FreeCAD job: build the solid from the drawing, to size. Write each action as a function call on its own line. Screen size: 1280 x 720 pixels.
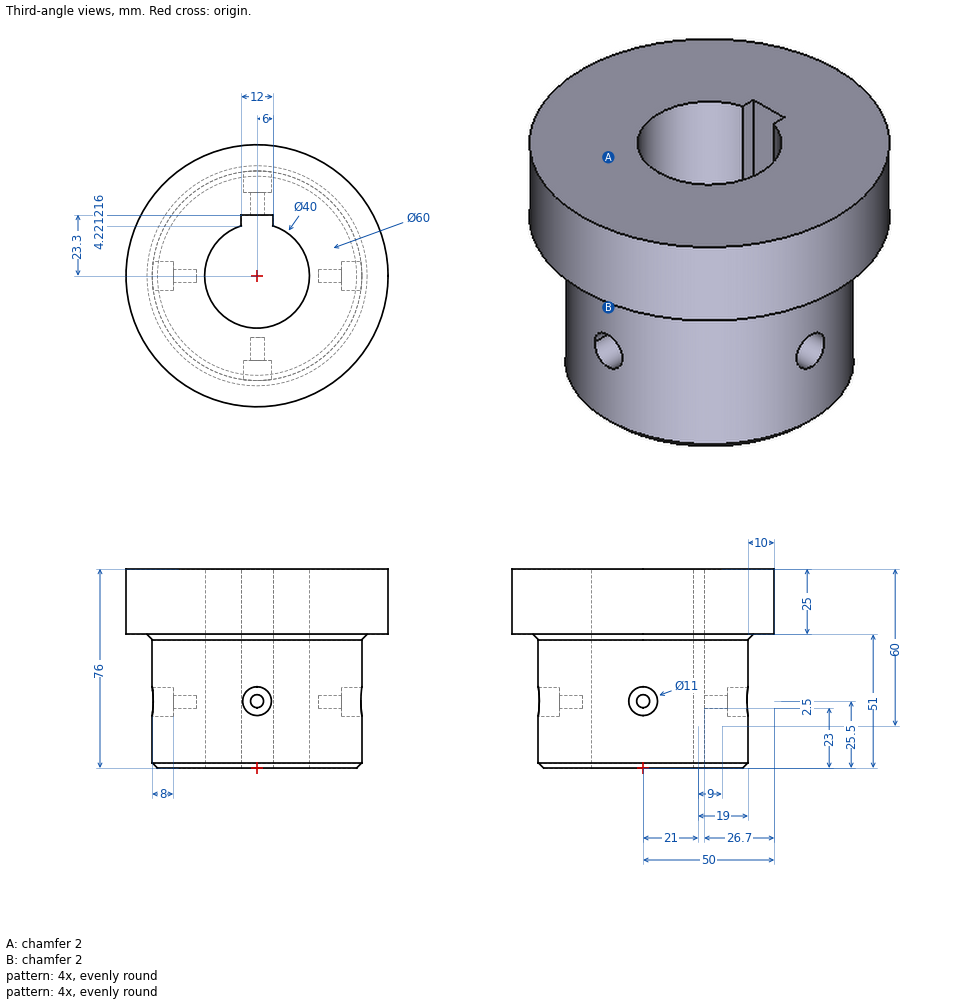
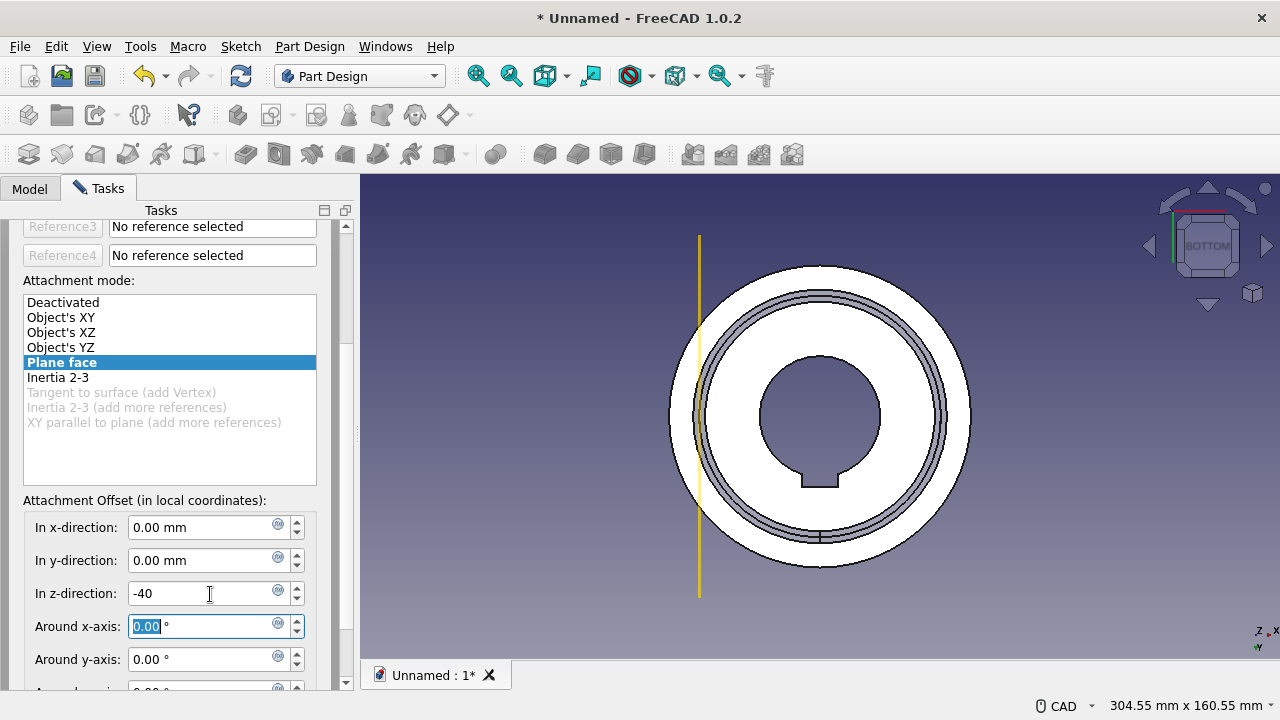
scroll(346, 455, up, 4)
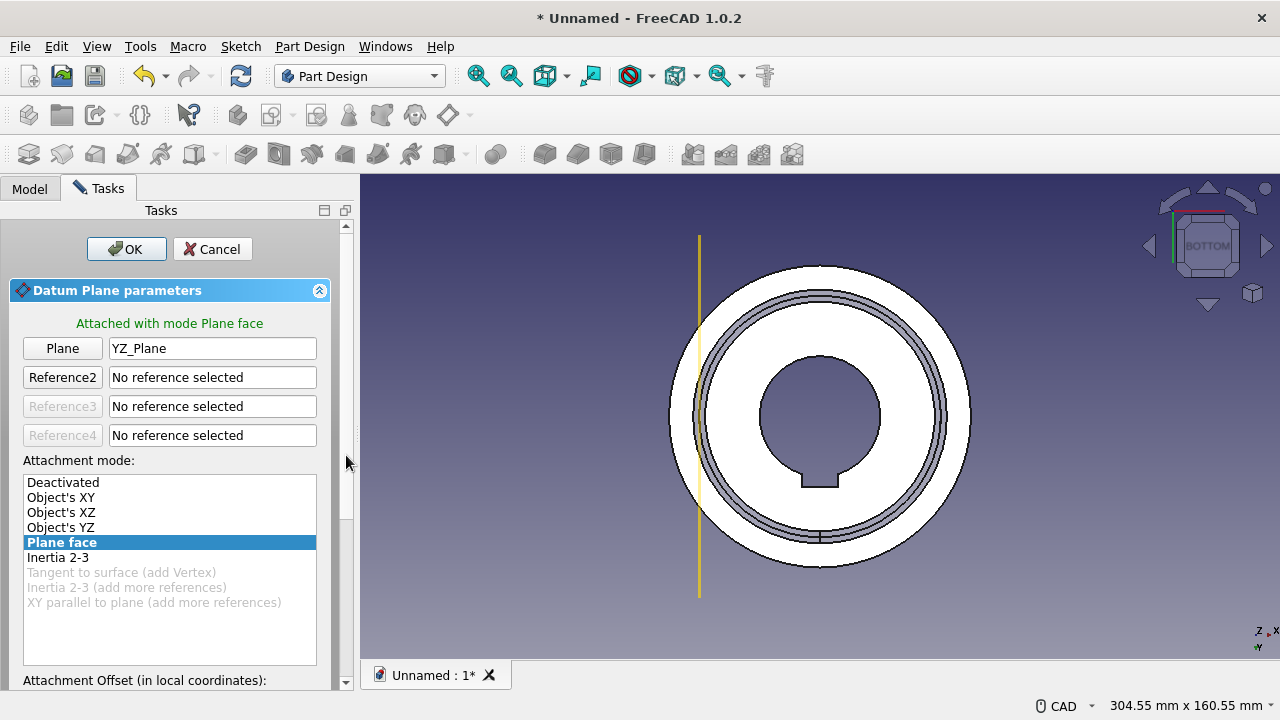
click(127, 249)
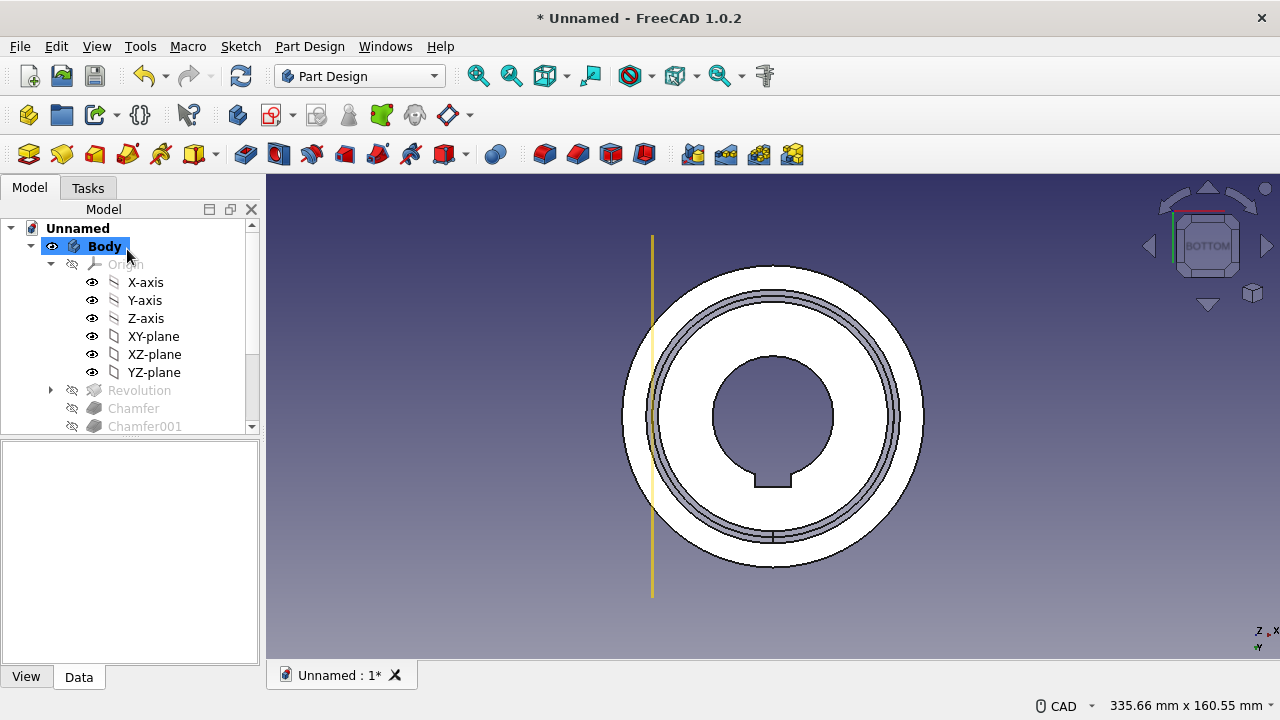
scroll(101, 332, down, 3)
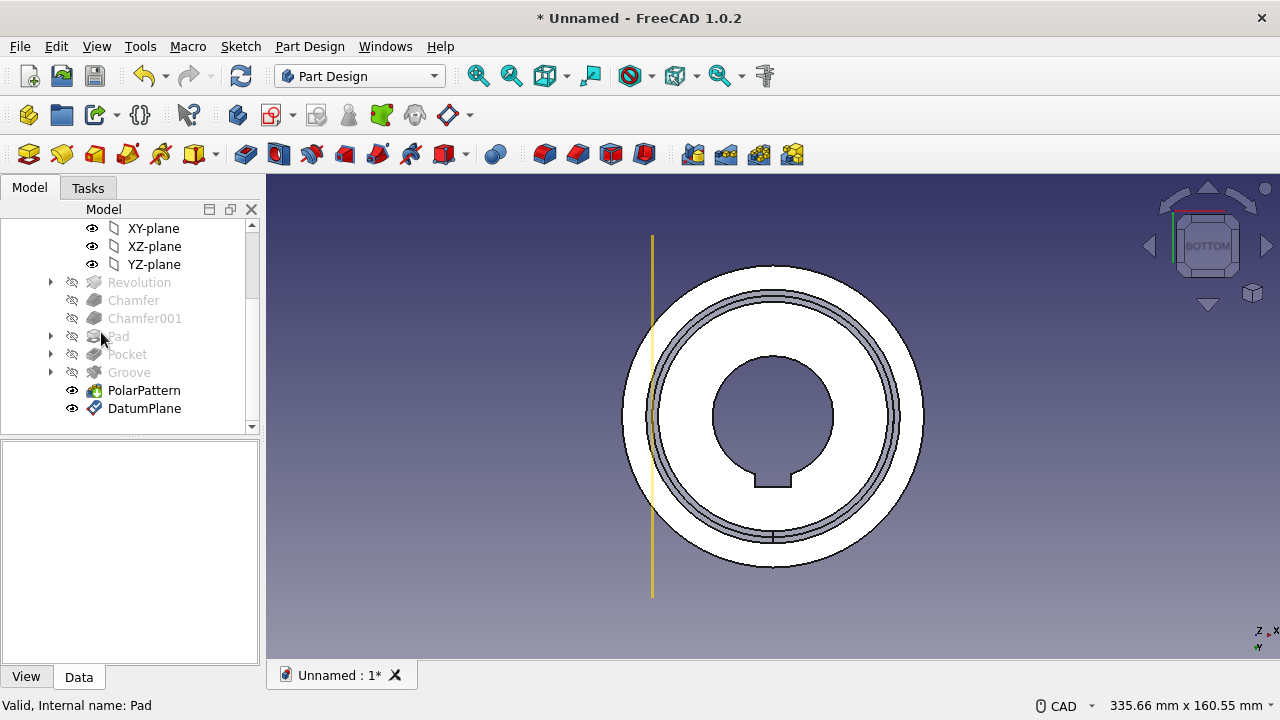
click(117, 408)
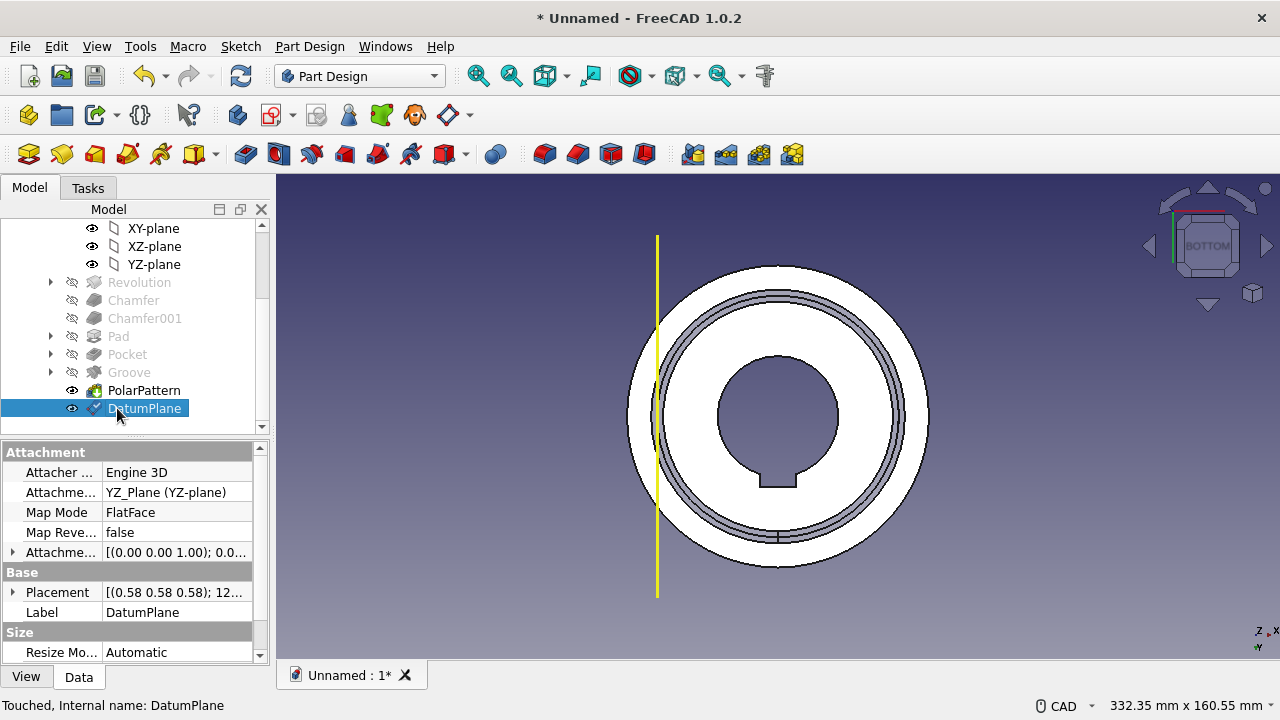
click(270, 116)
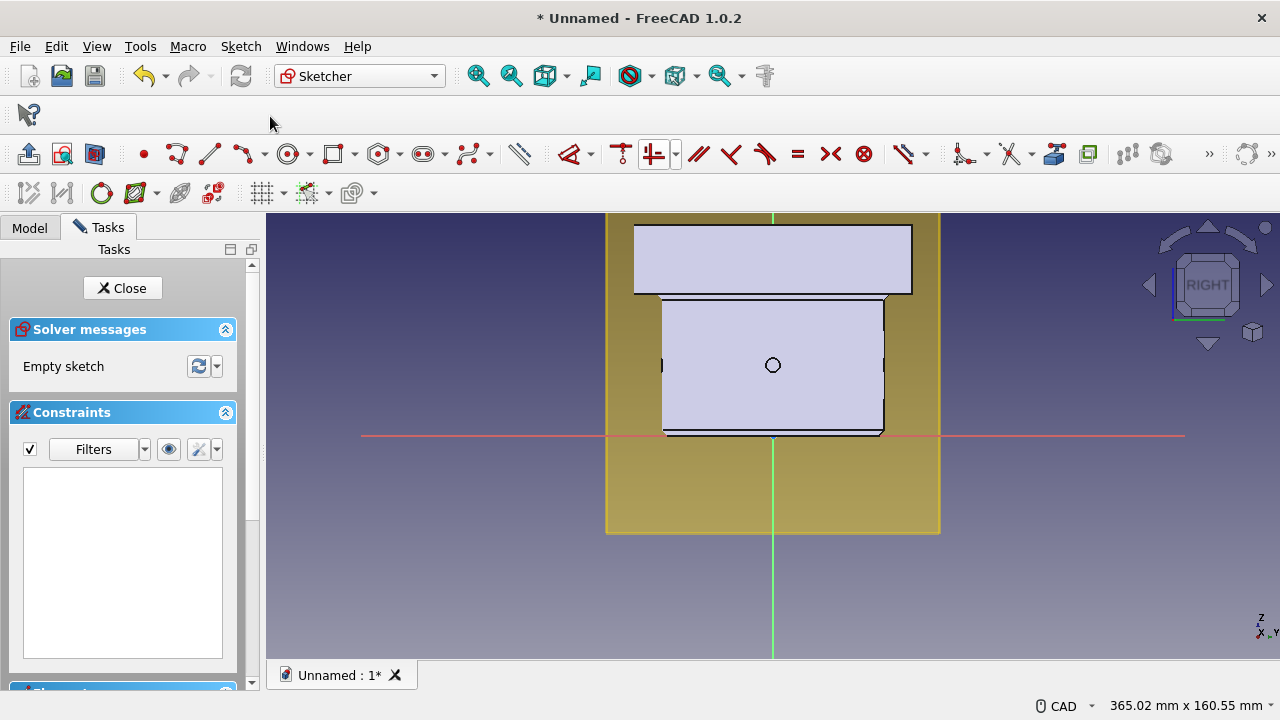
key(q)
key(s)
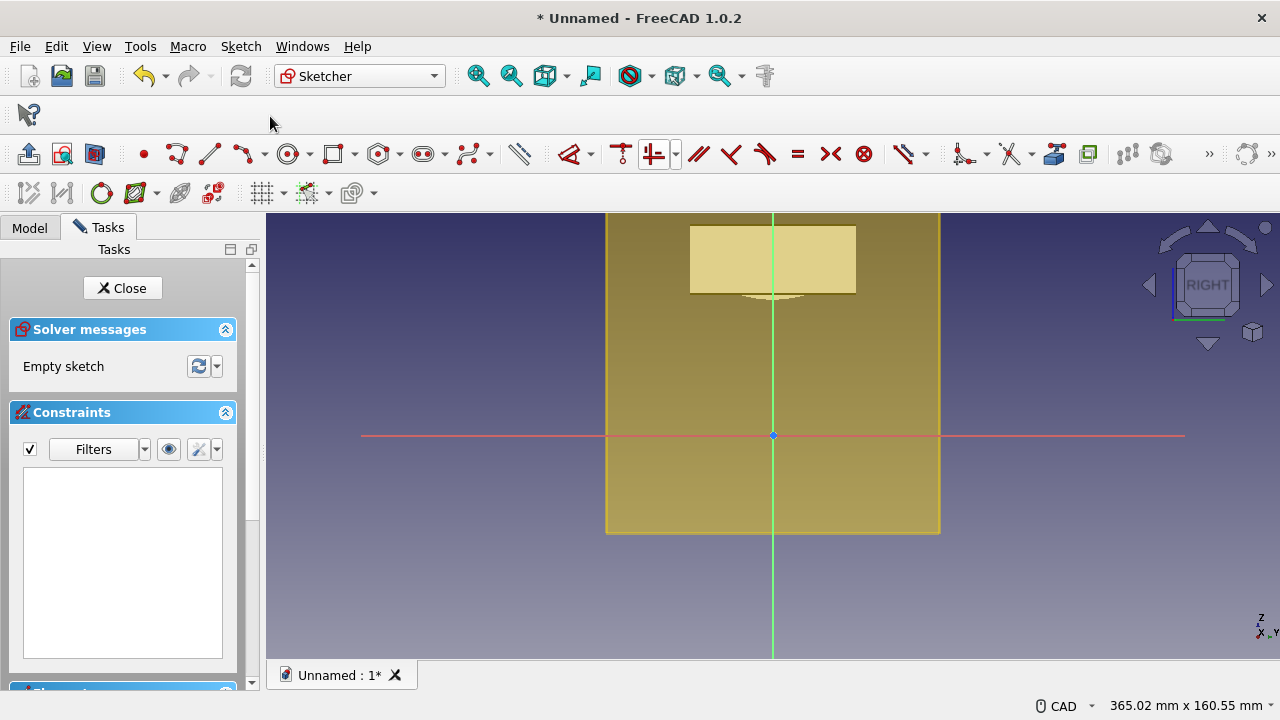
scroll(782, 356, up, 11)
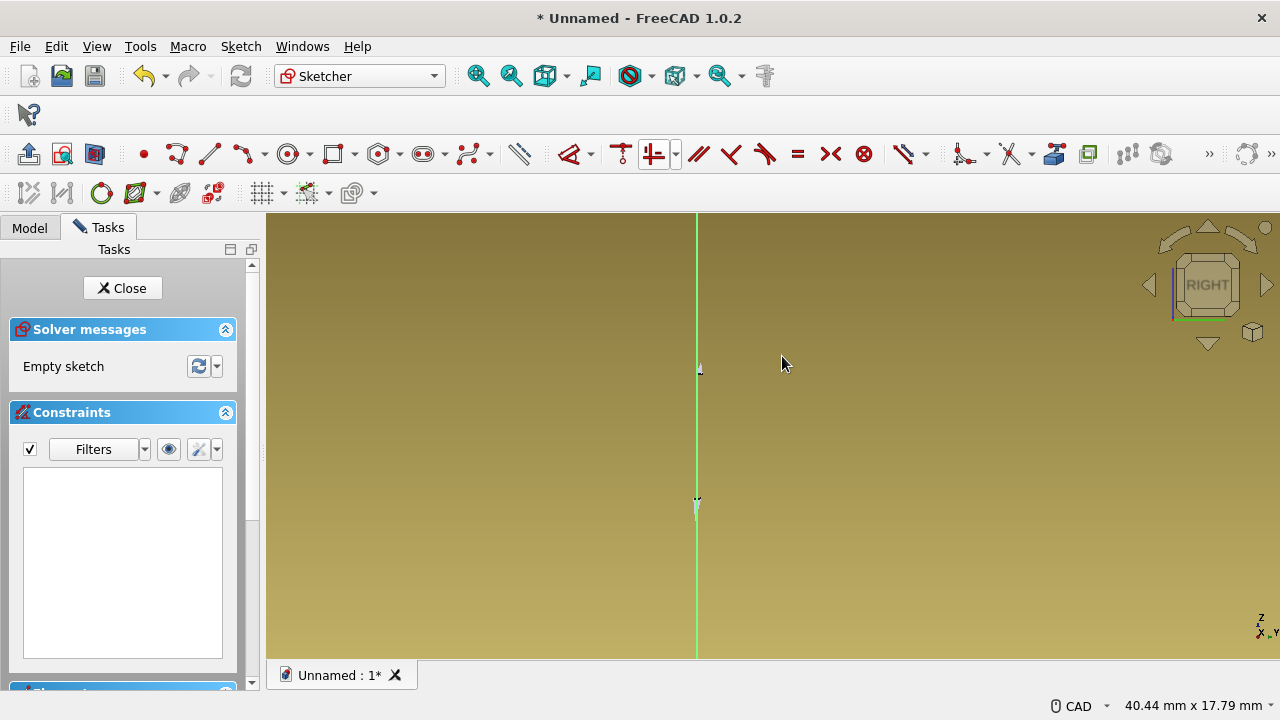
key(g)
key(c)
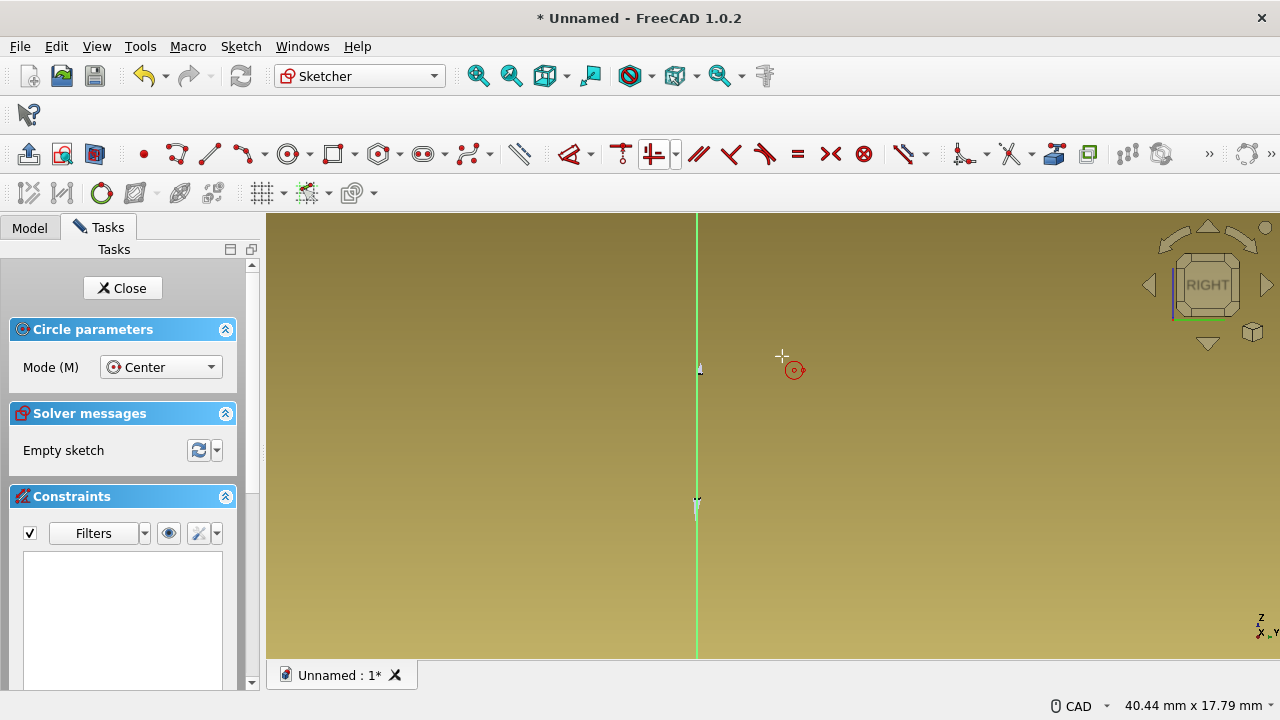
click(697, 436)
move(794, 339)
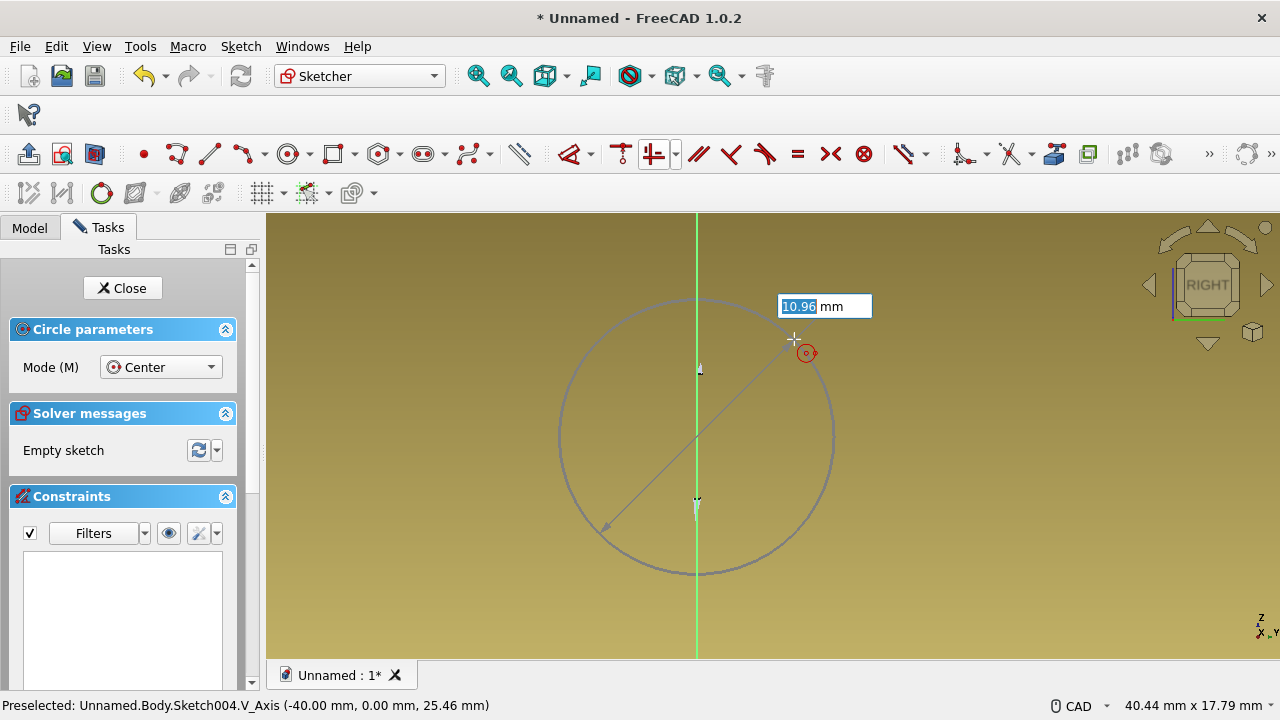
text(11)
key(Return)
key(Escape)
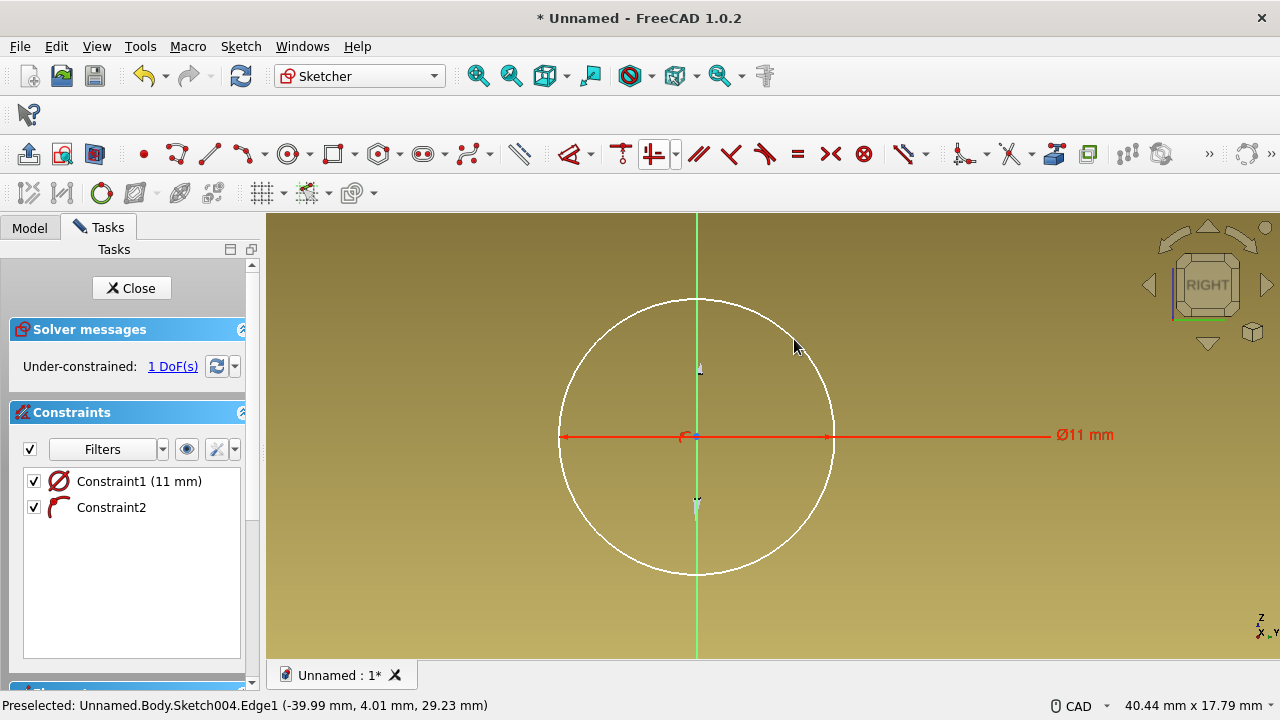
click(568, 154)